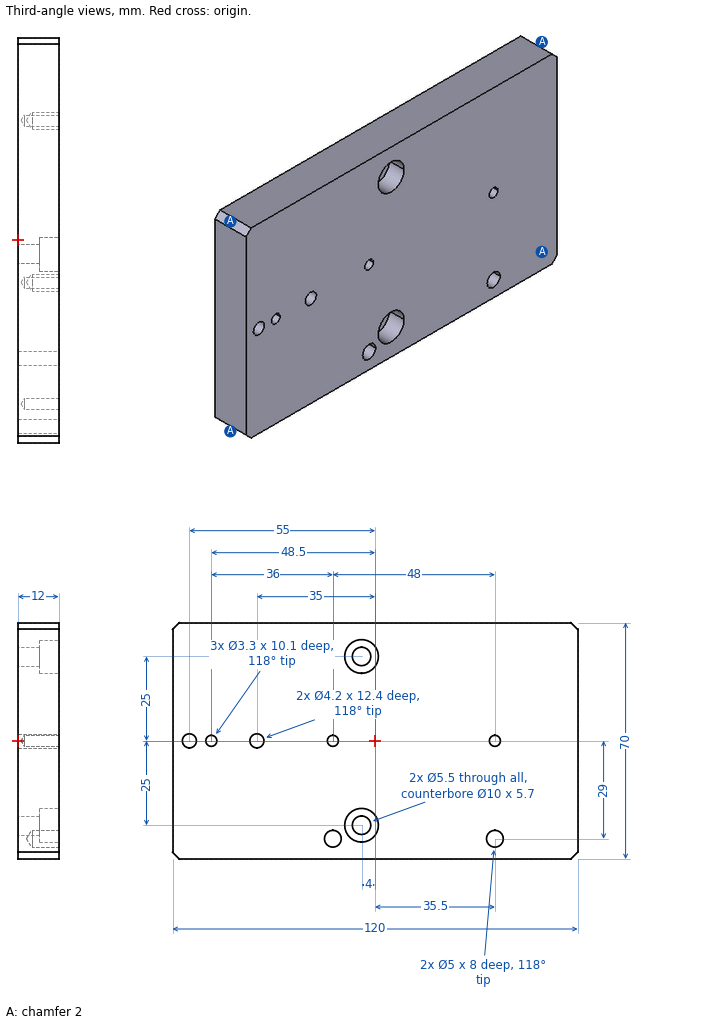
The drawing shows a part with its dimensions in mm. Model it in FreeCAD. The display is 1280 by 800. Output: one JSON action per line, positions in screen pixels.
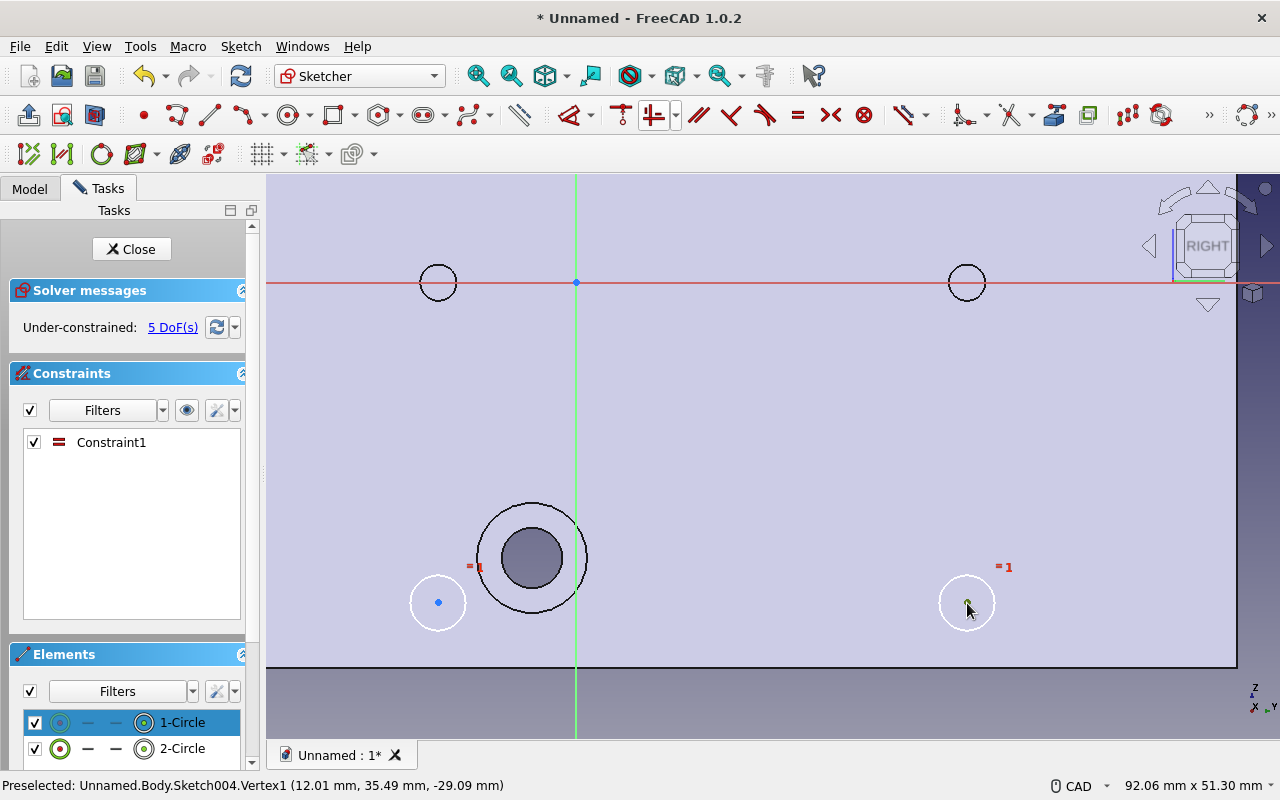
{"action": "left_click", "coordinate": [438, 603]}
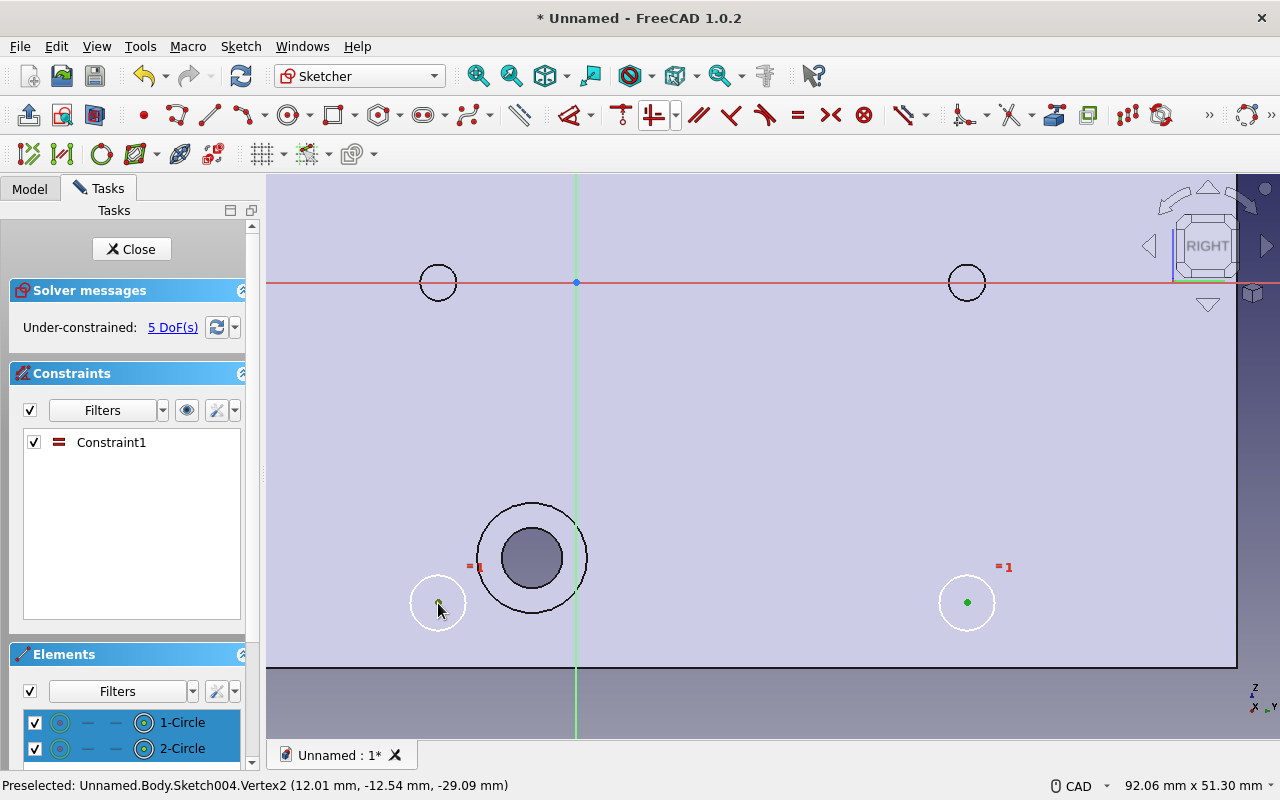
{"action": "left_click", "coordinate": [676, 116]}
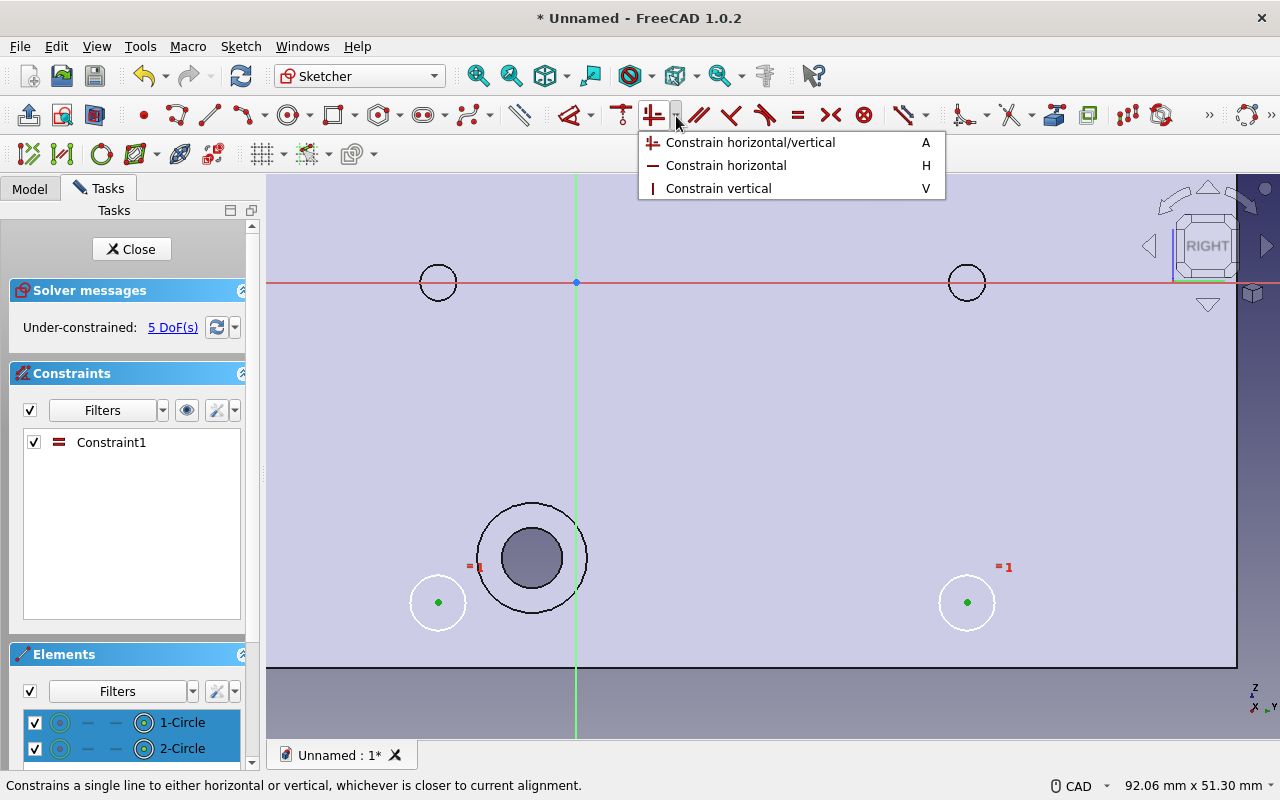
{"action": "left_click", "coordinate": [792, 166]}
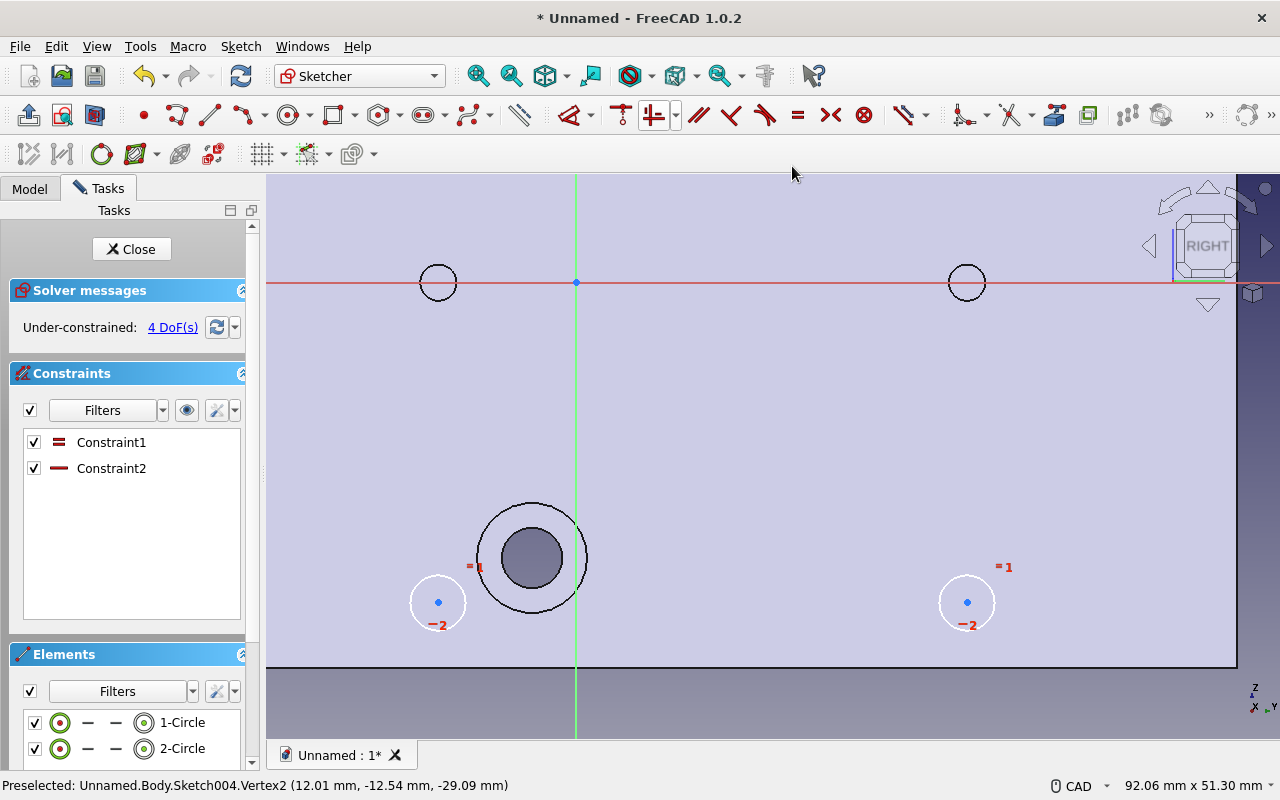
{"action": "left_click", "coordinate": [568, 116]}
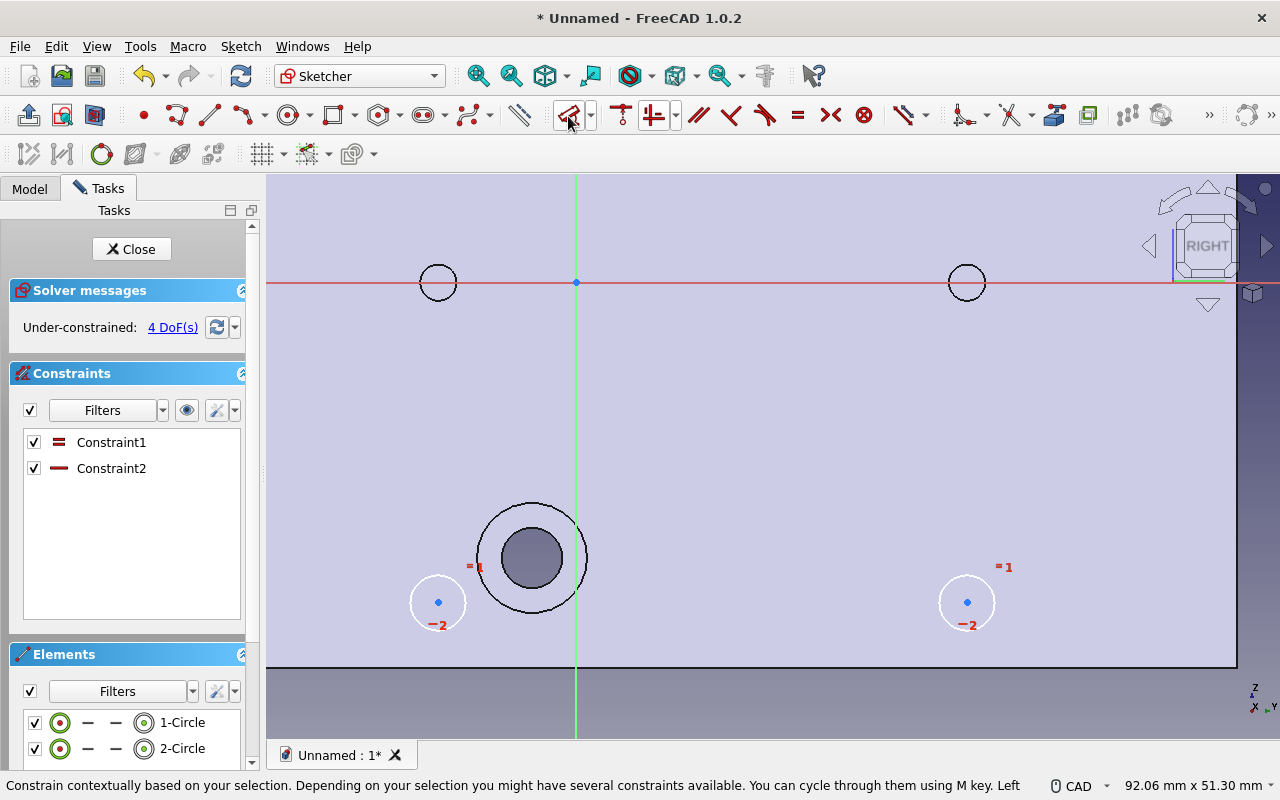
{"action": "left_click", "coordinate": [986, 583]}
{"action": "left_click", "coordinate": [1008, 560]}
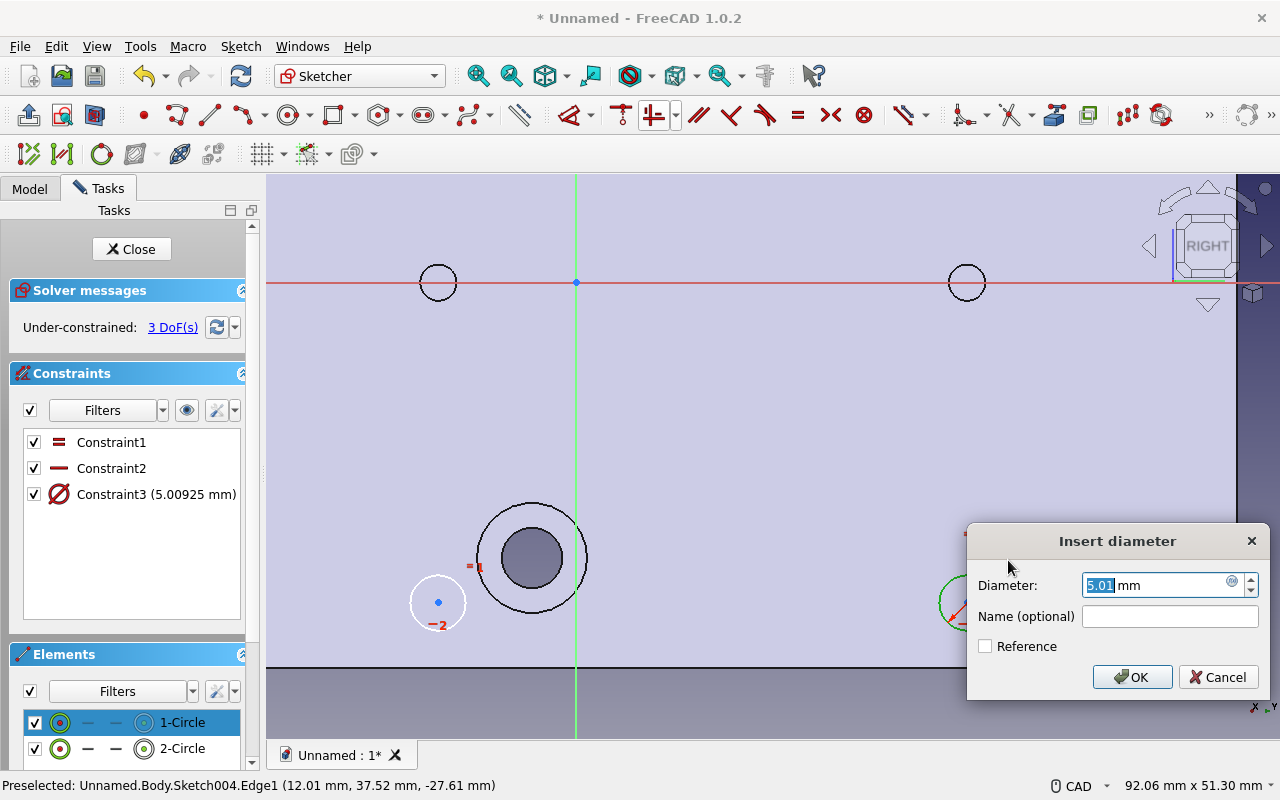
{"action": "type", "text": "5"}
{"action": "key", "text": "Return"}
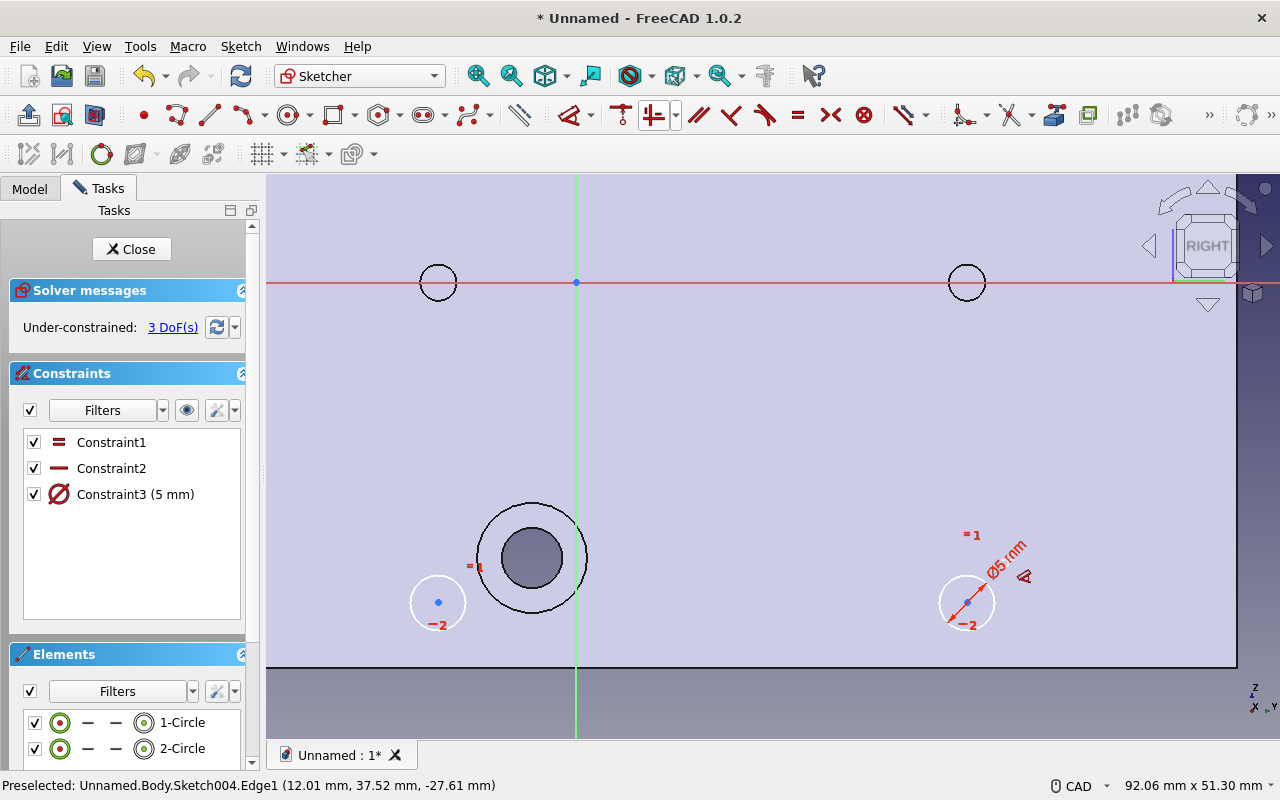
{"action": "left_click", "coordinate": [967, 603]}
{"action": "left_click", "coordinate": [1001, 443]}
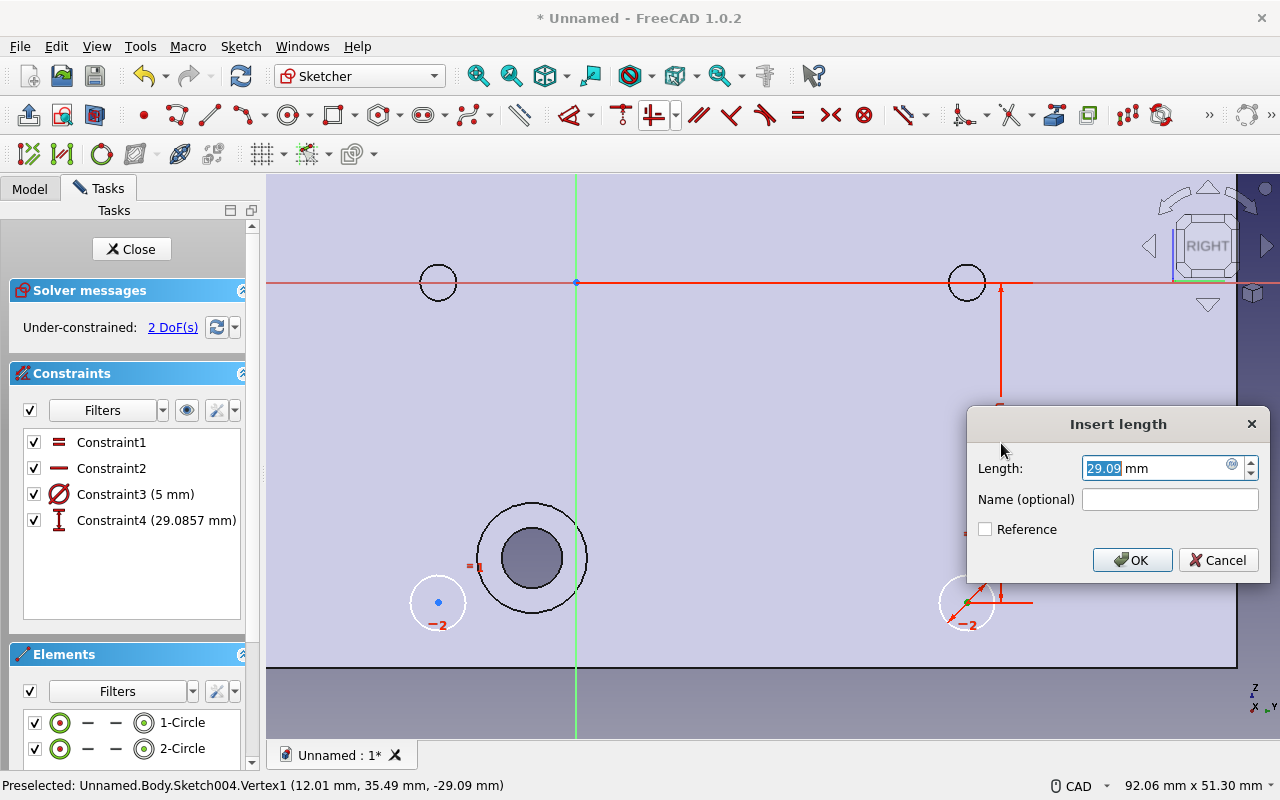
{"action": "type", "text": "29"}
{"action": "key", "text": "Return"}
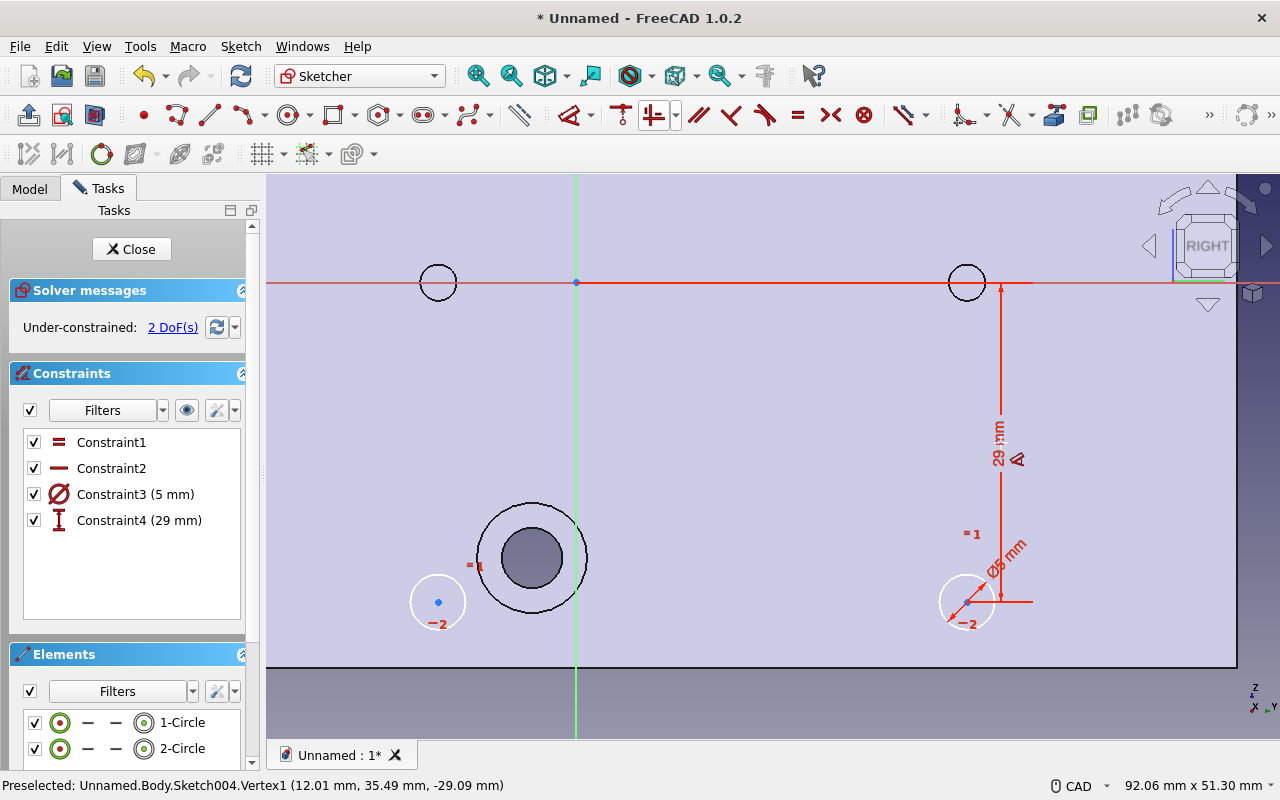
{"action": "left_click", "coordinate": [967, 602]}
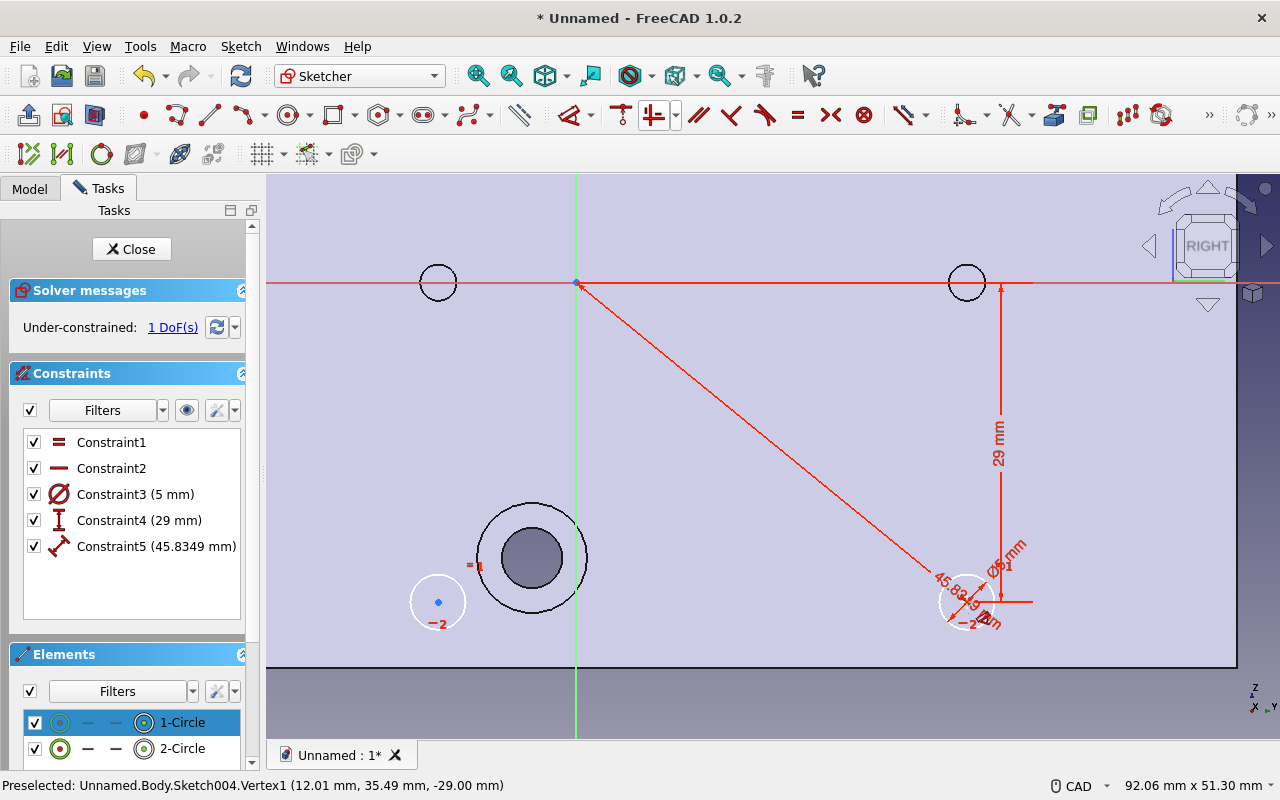
{"action": "left_click", "coordinate": [438, 602]}
{"action": "left_click", "coordinate": [702, 636]}